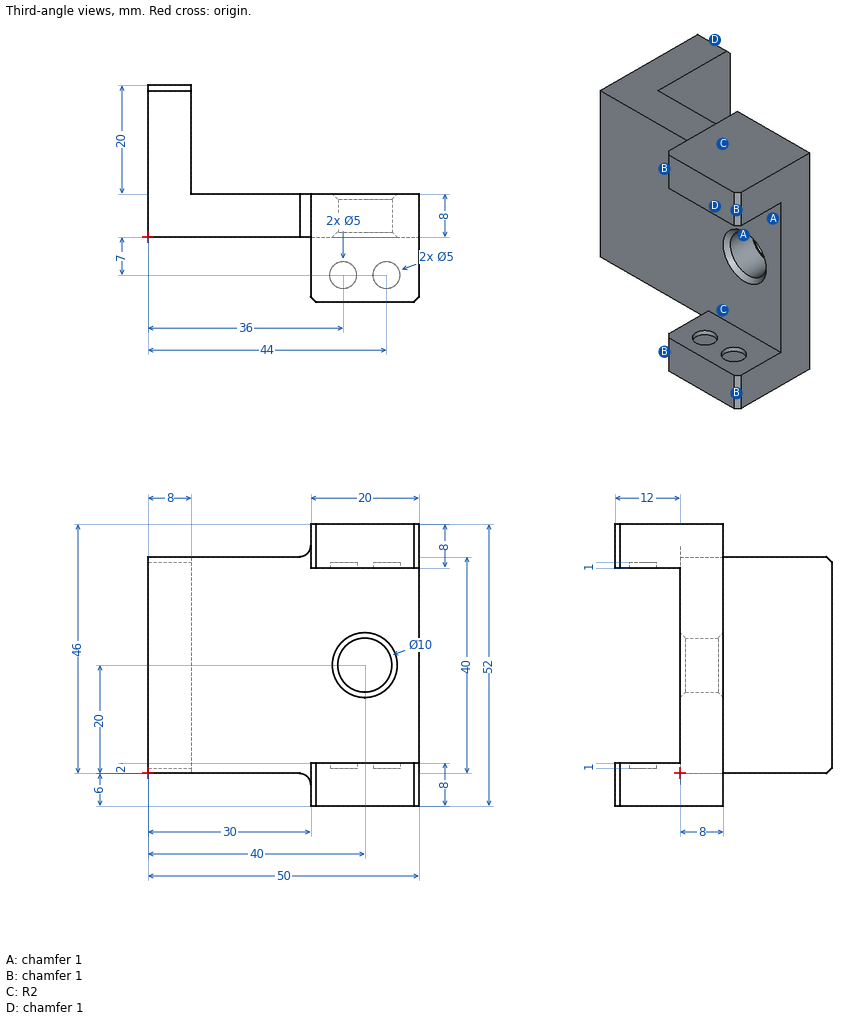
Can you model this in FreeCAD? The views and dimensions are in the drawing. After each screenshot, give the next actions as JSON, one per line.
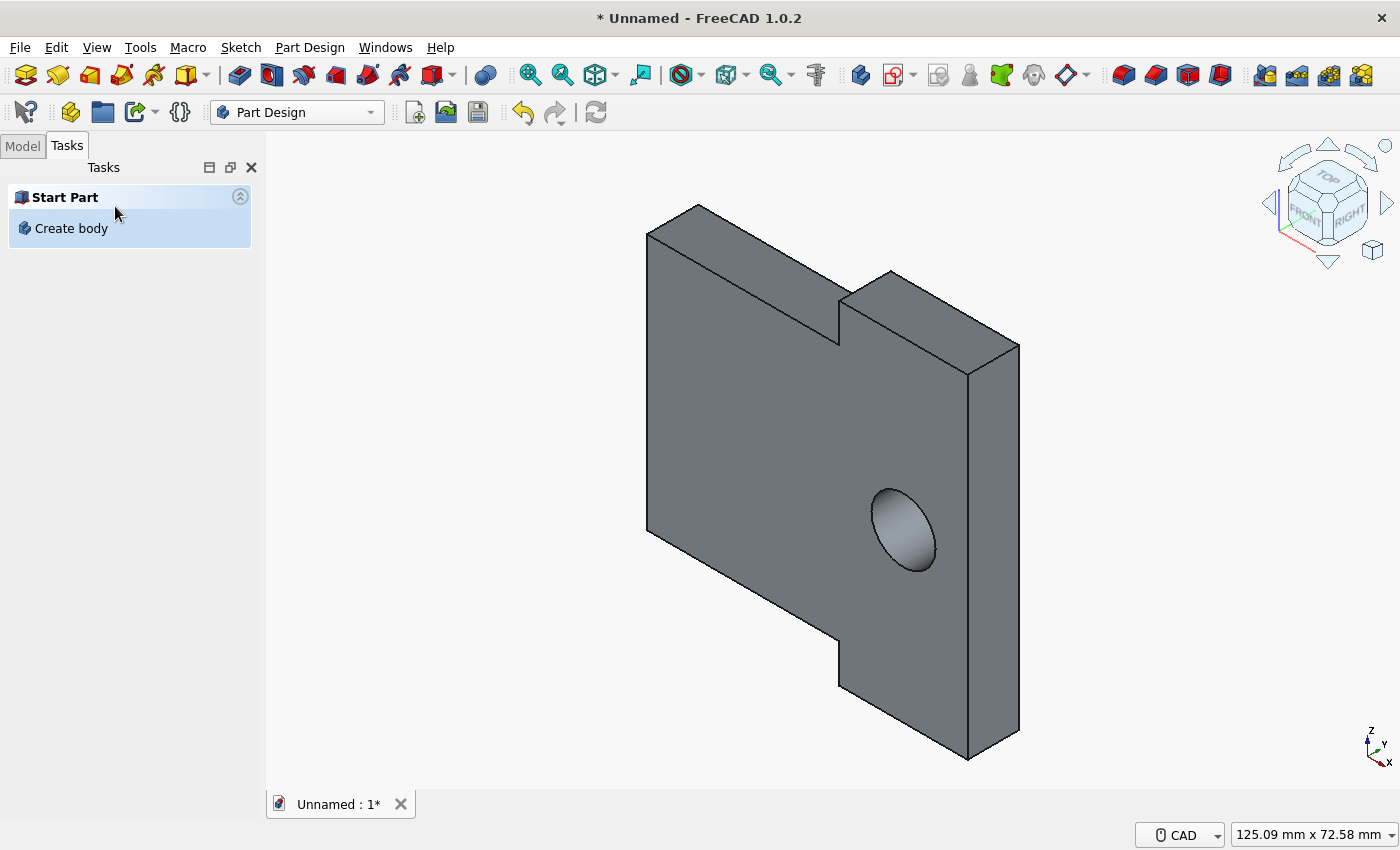
{"action": "left_click", "coordinate": [871, 511]}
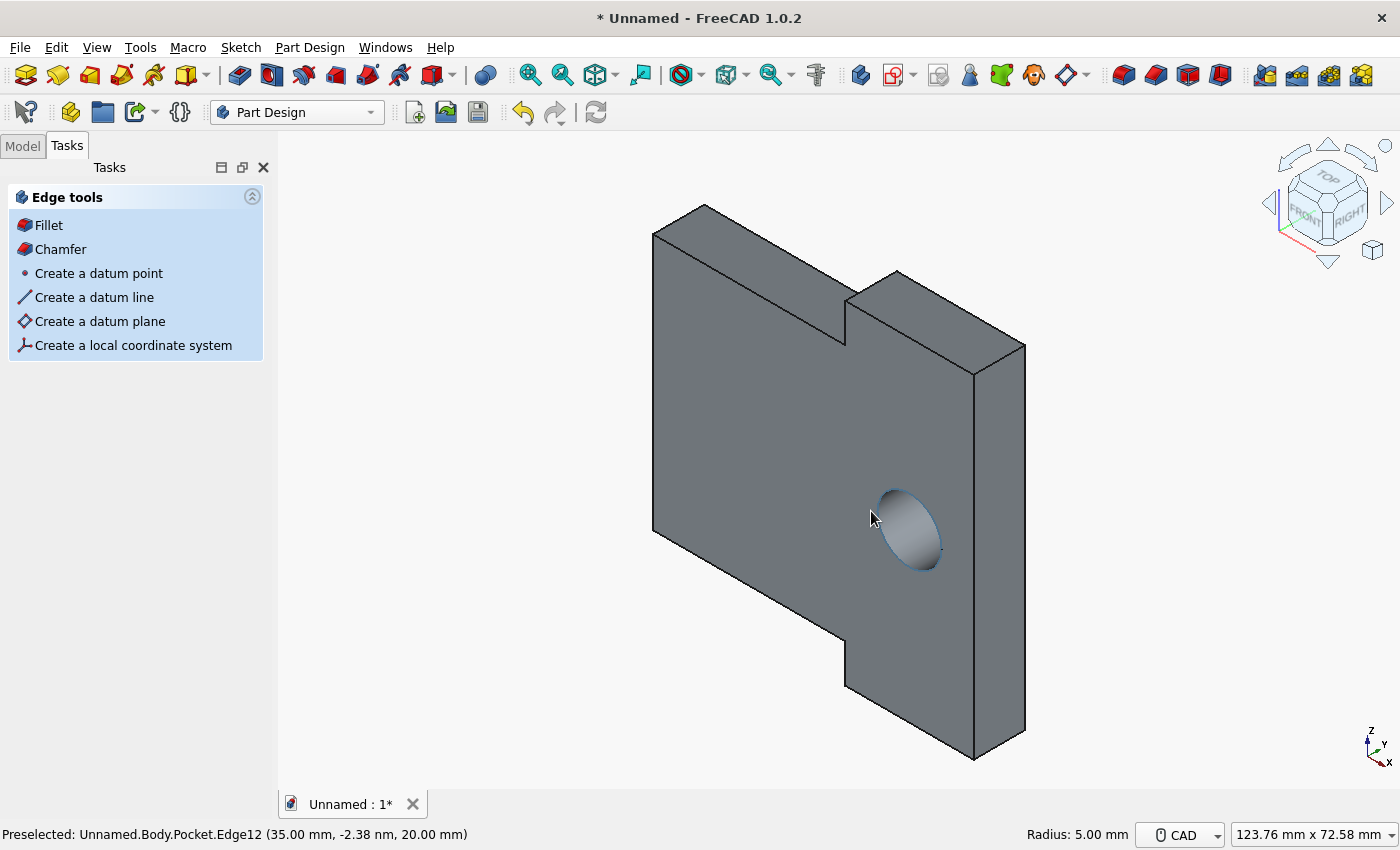
{"action": "key", "text": "2"}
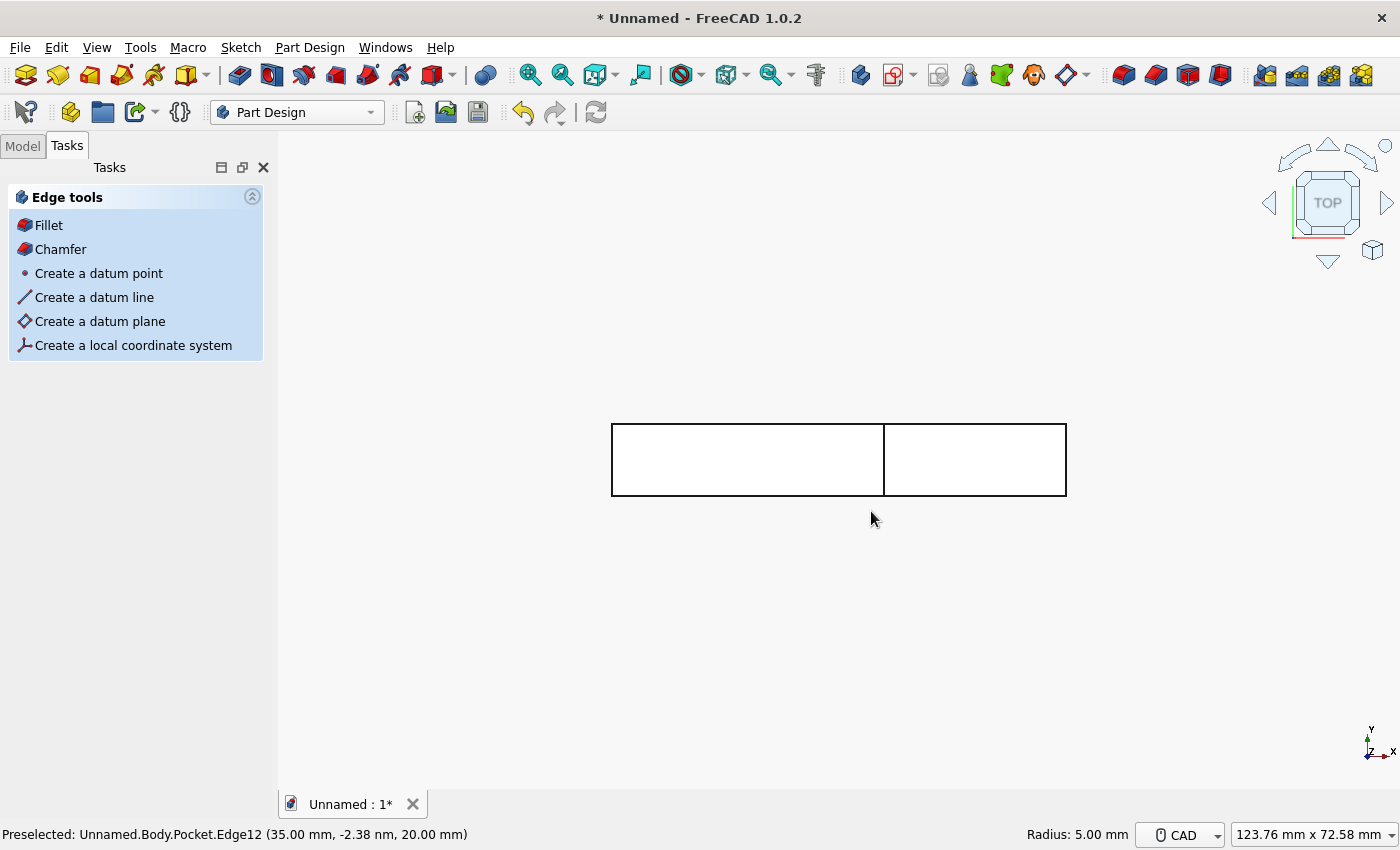
{"action": "left_click", "coordinate": [532, 76]}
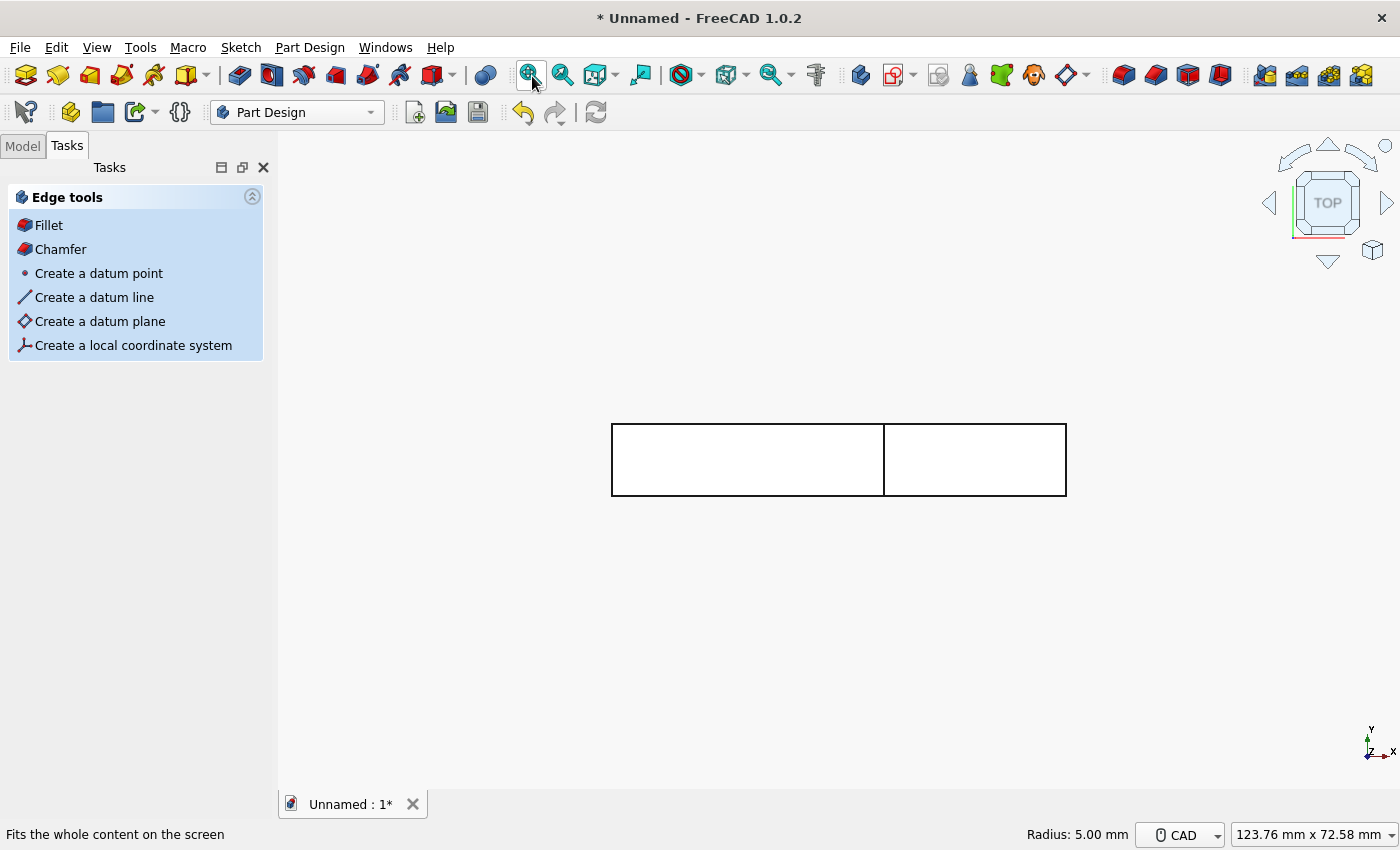
{"action": "key", "text": "0"}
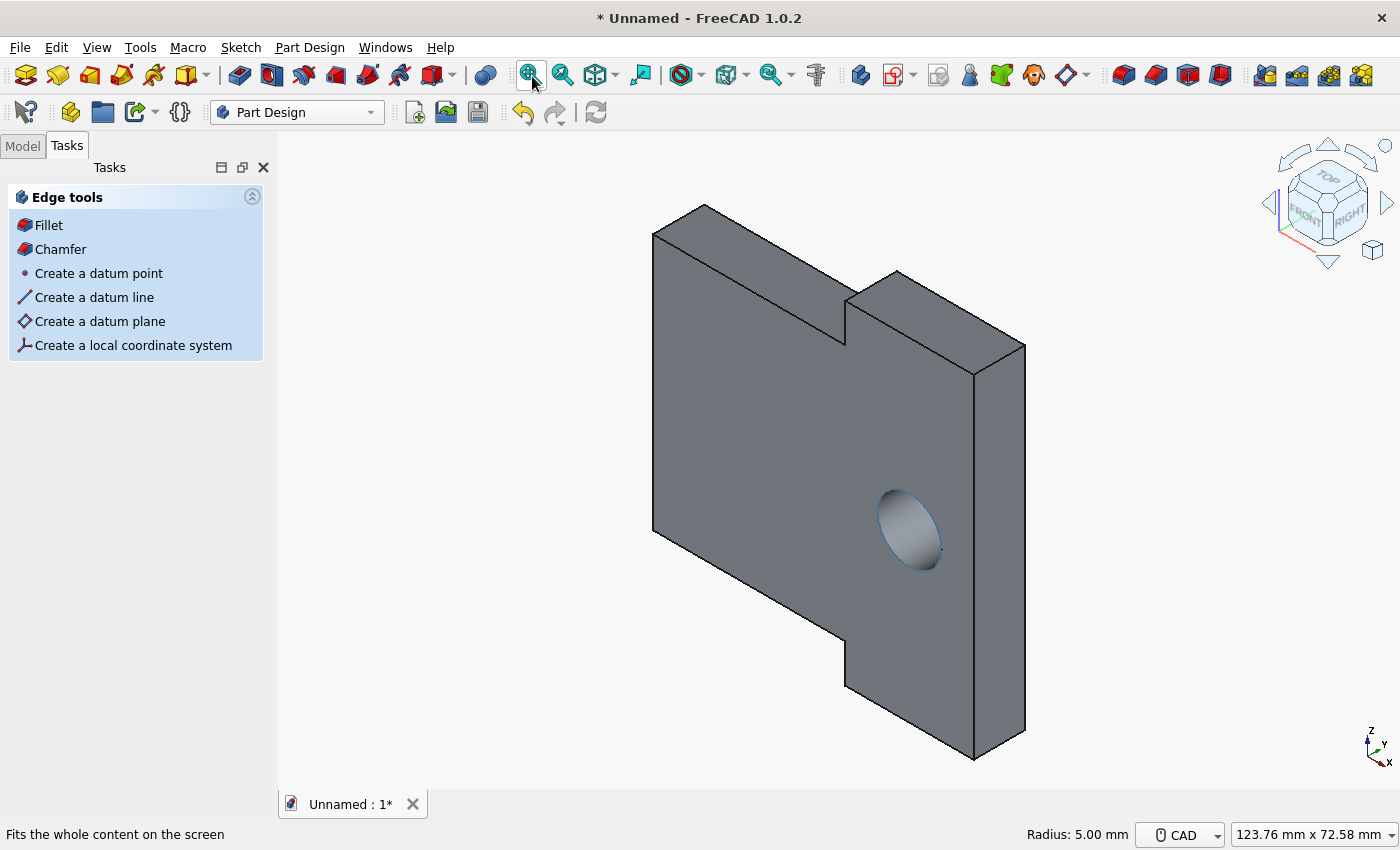
{"action": "key", "text": "1"}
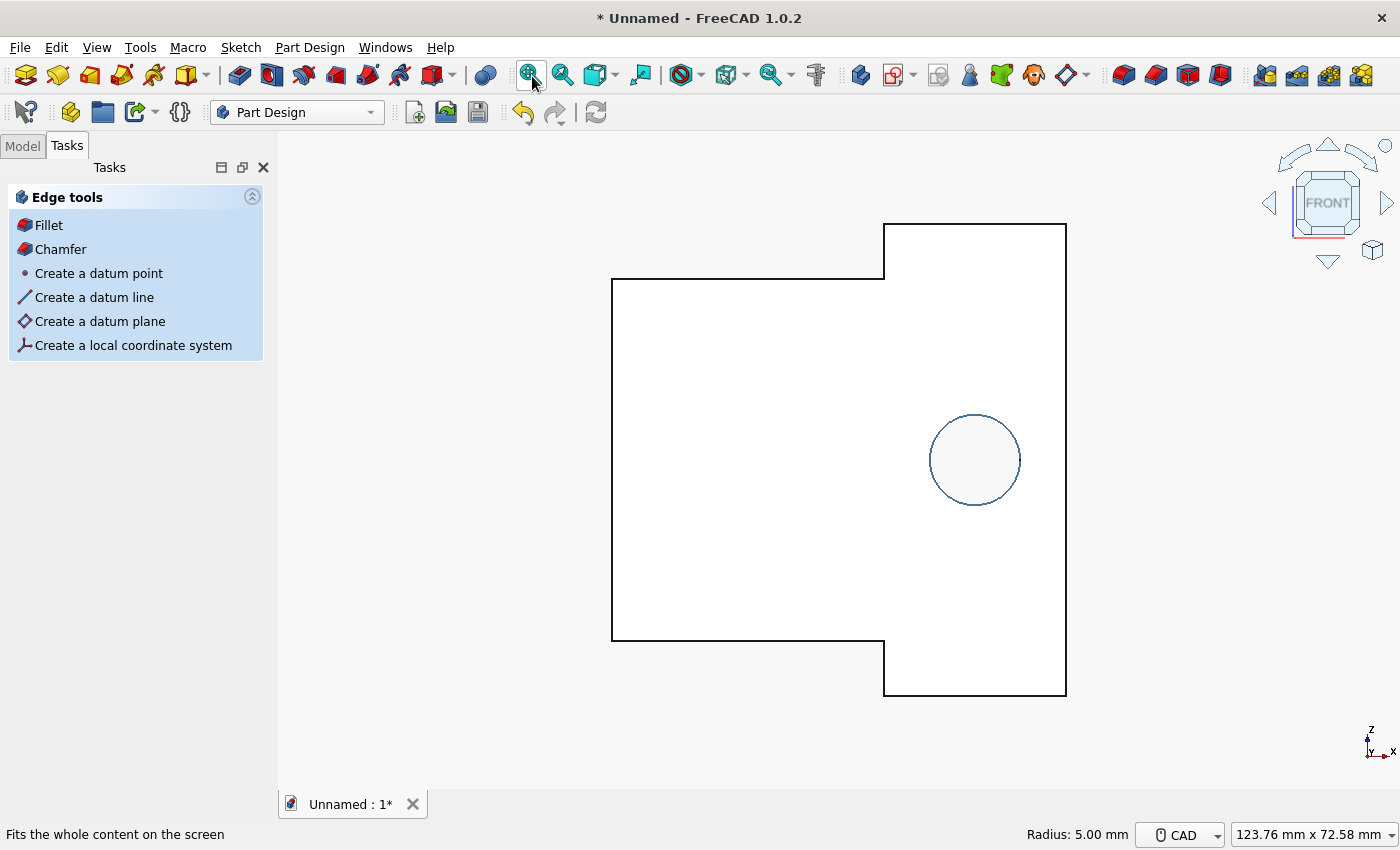
{"action": "key", "text": "3"}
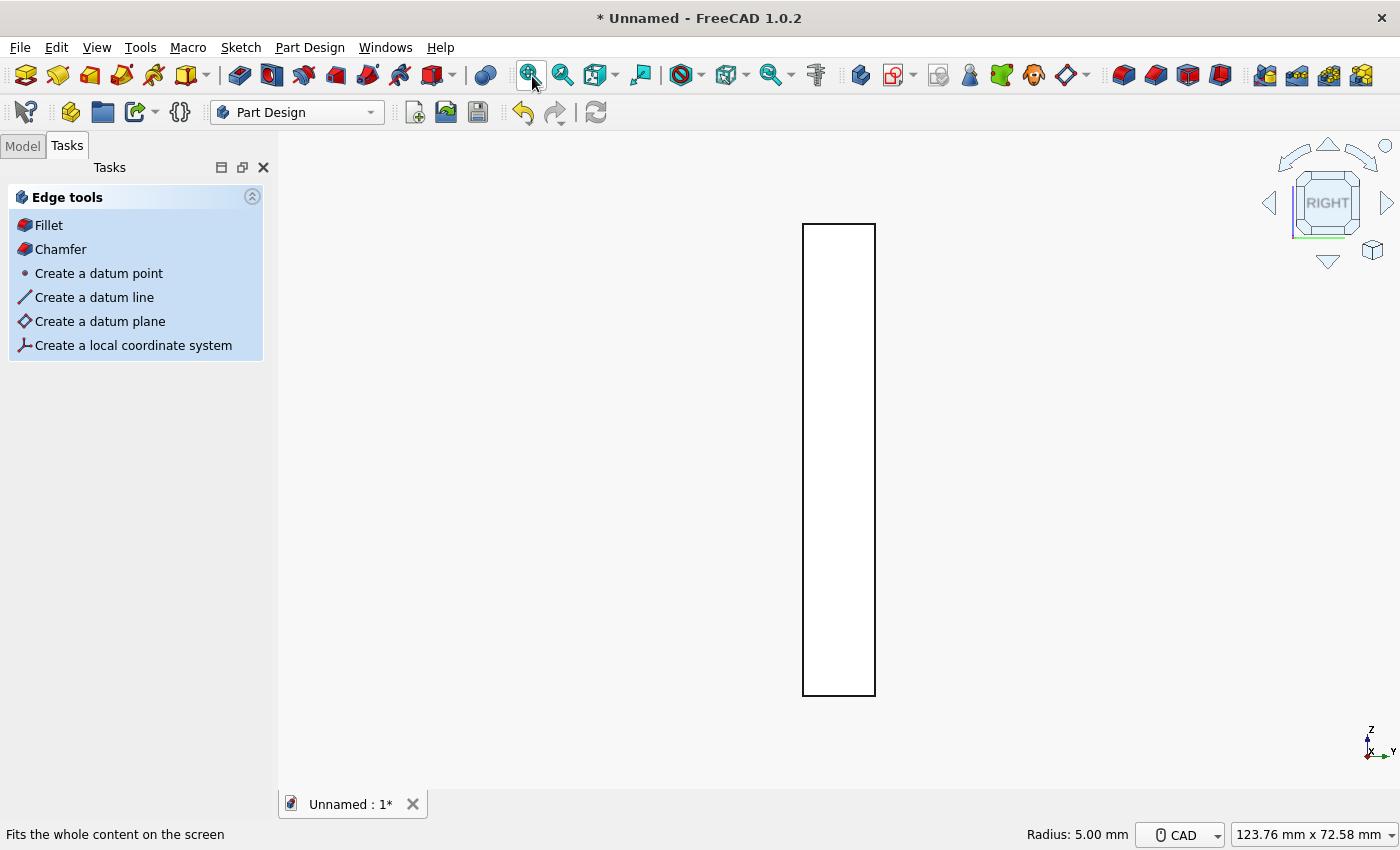
{"action": "key", "text": "5"}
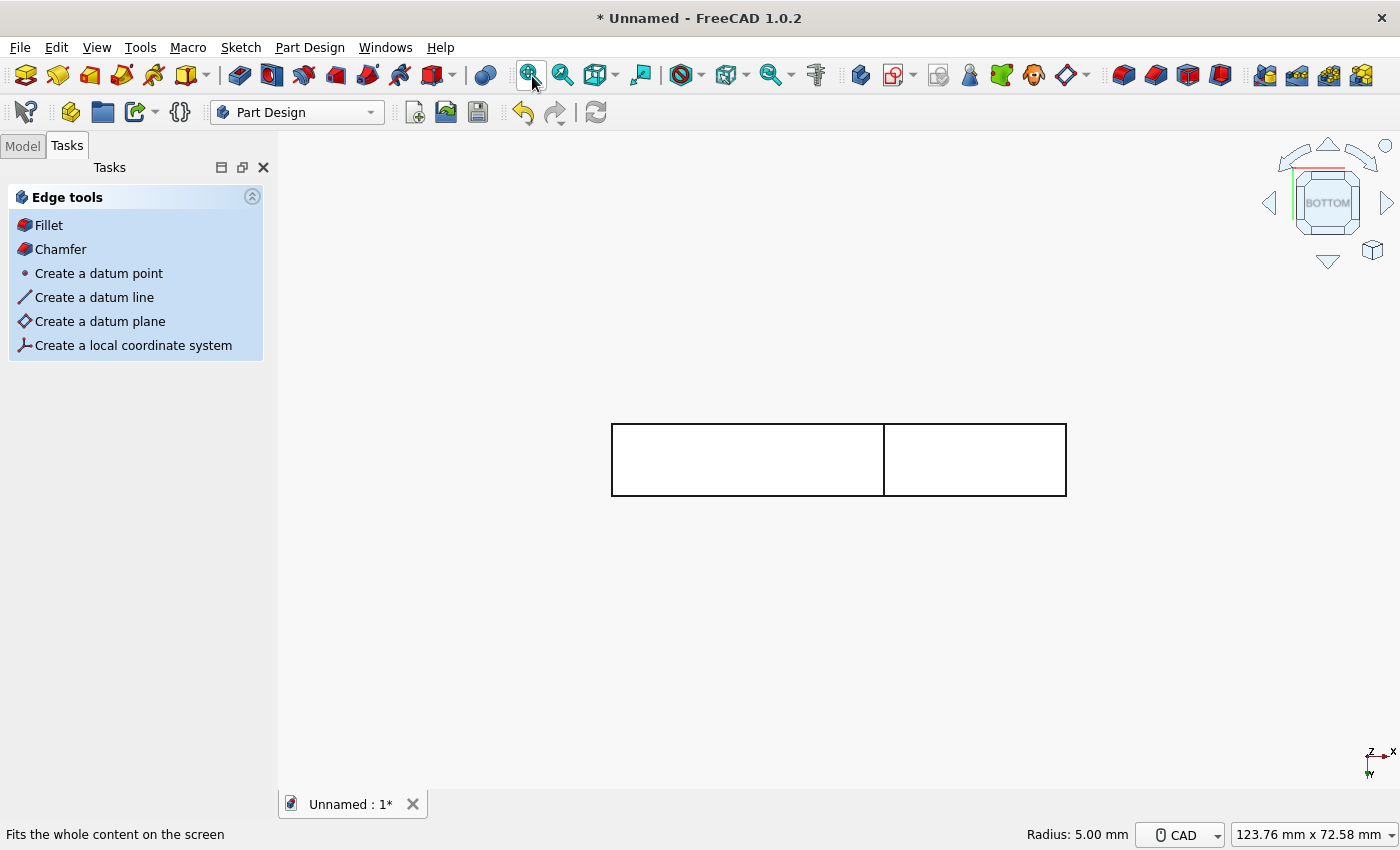
{"action": "key", "text": "v f"}